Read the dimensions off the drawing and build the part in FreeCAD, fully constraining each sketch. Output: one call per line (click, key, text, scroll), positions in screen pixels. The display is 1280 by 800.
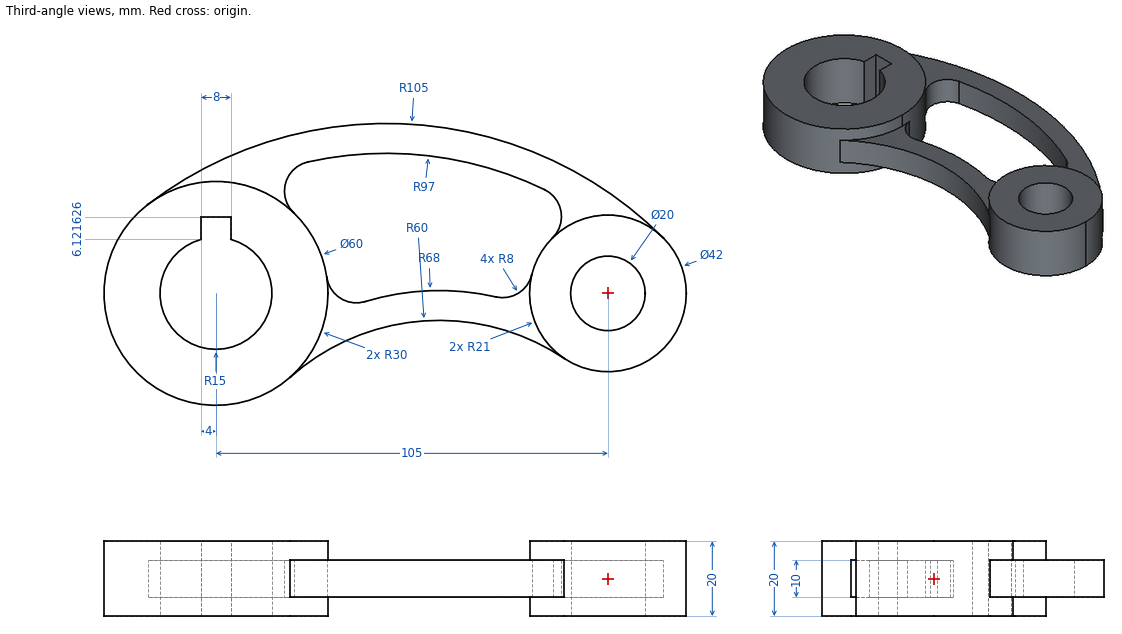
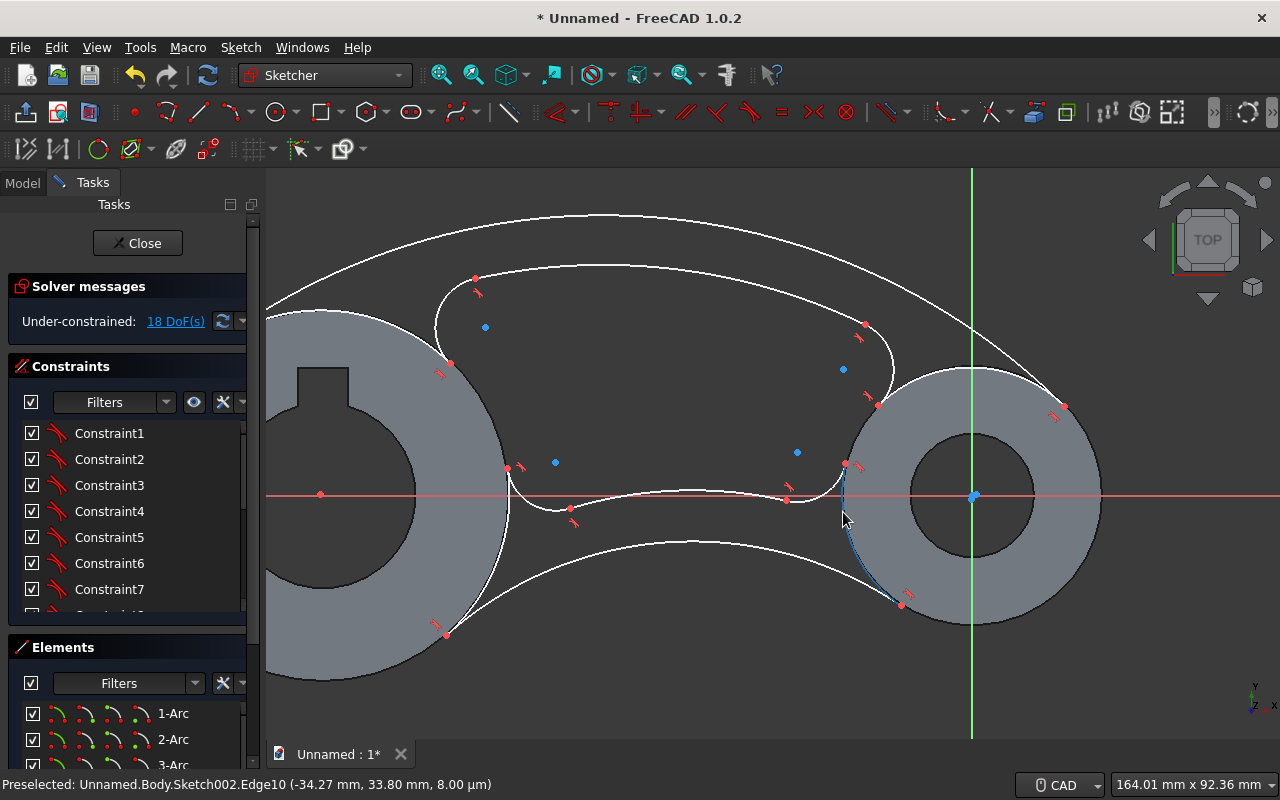
click(843, 512)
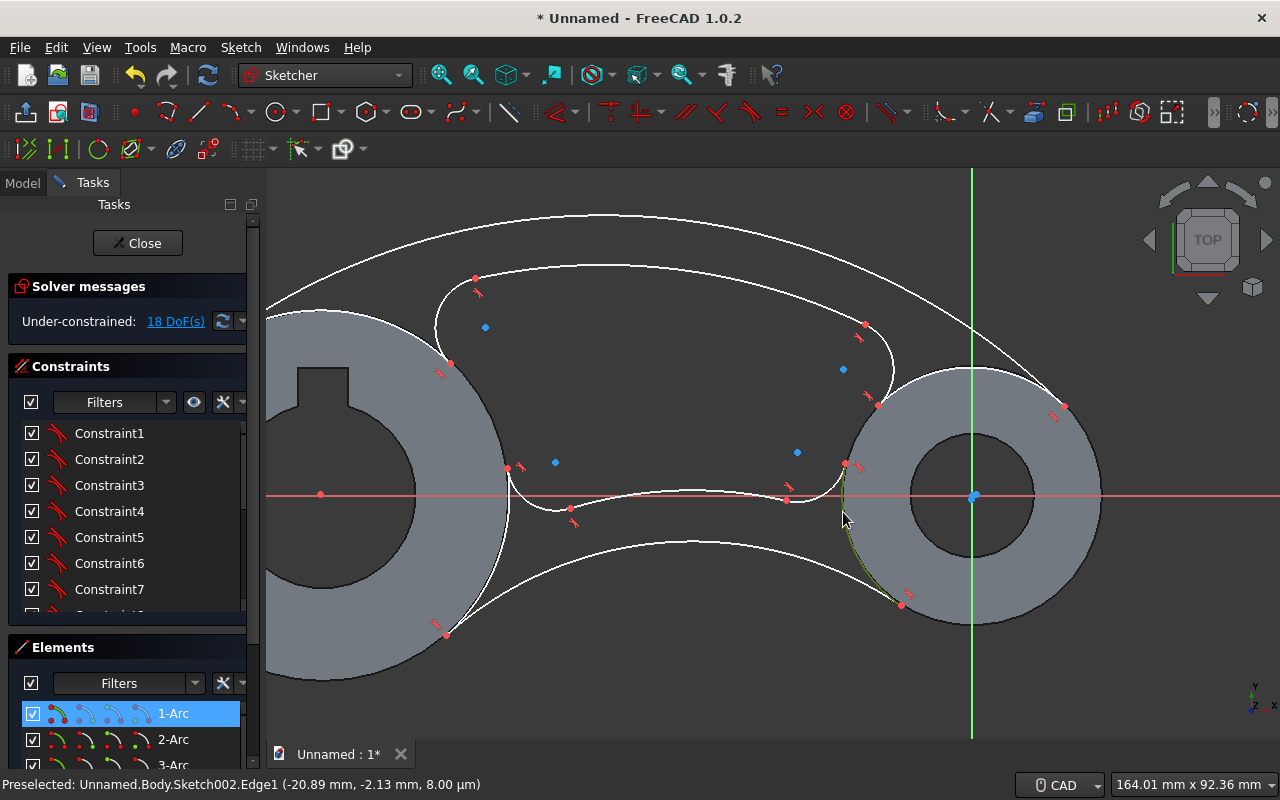
click(1012, 374)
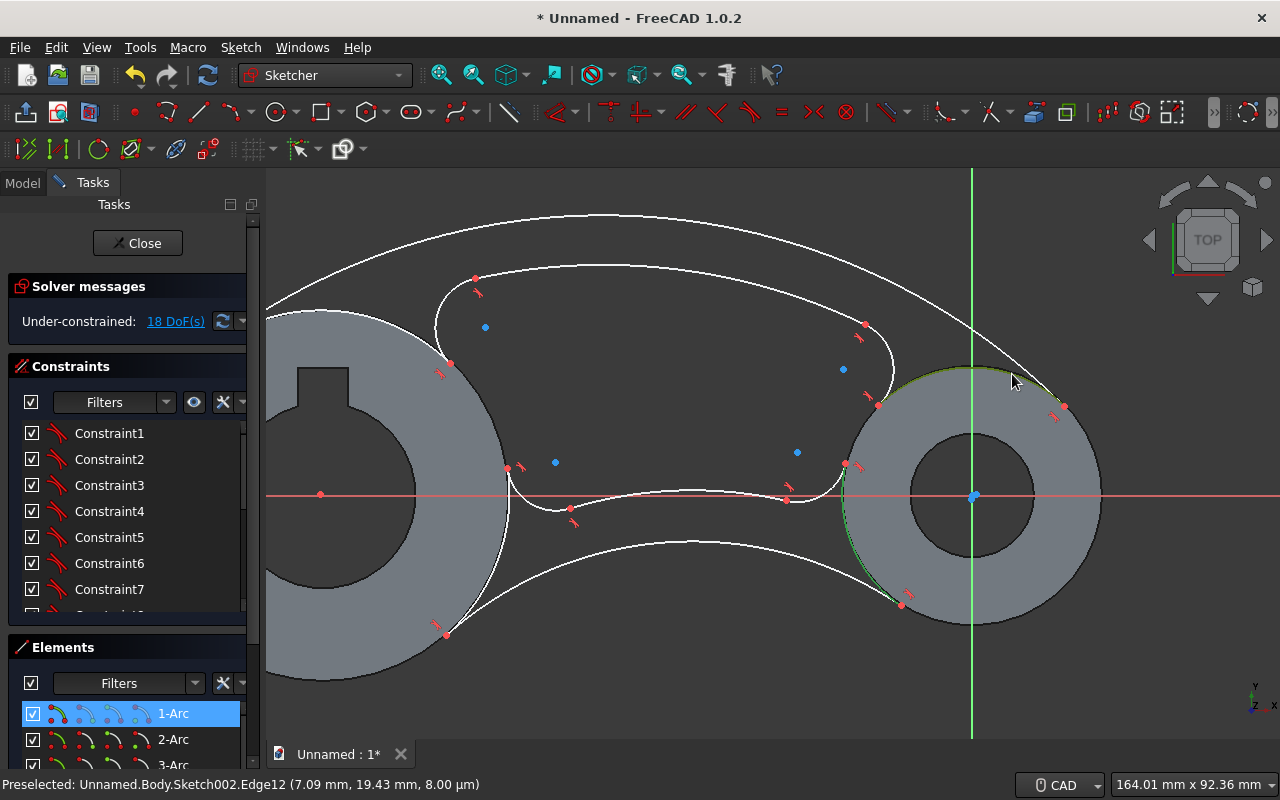
key(c)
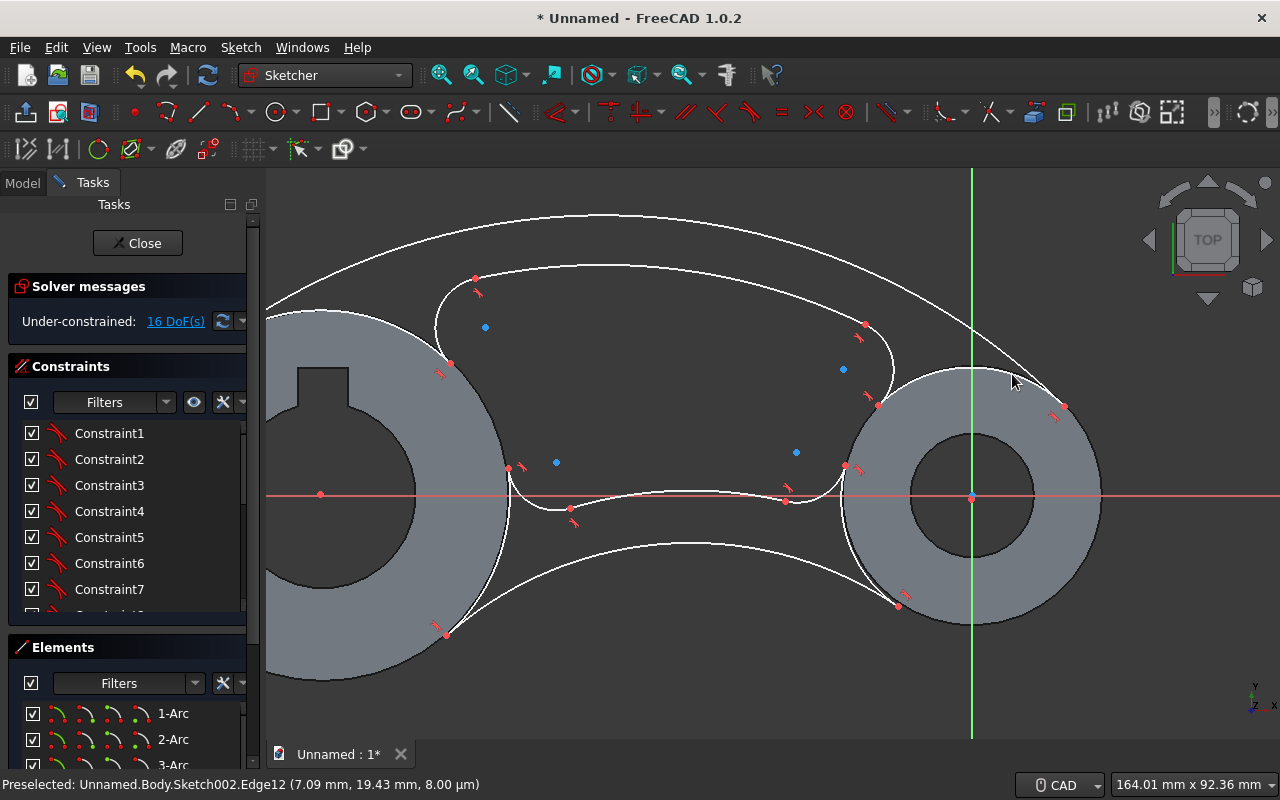
drag(961, 486, 982, 509)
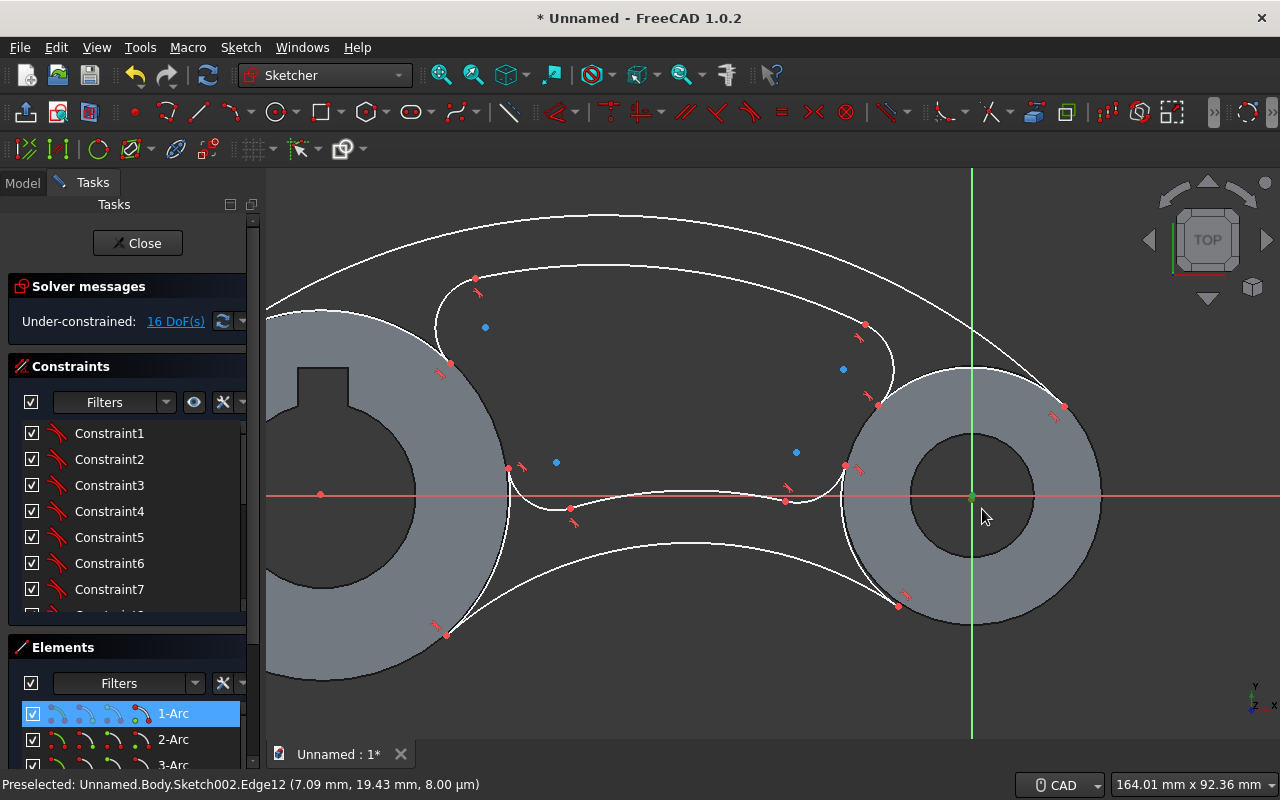
key(c)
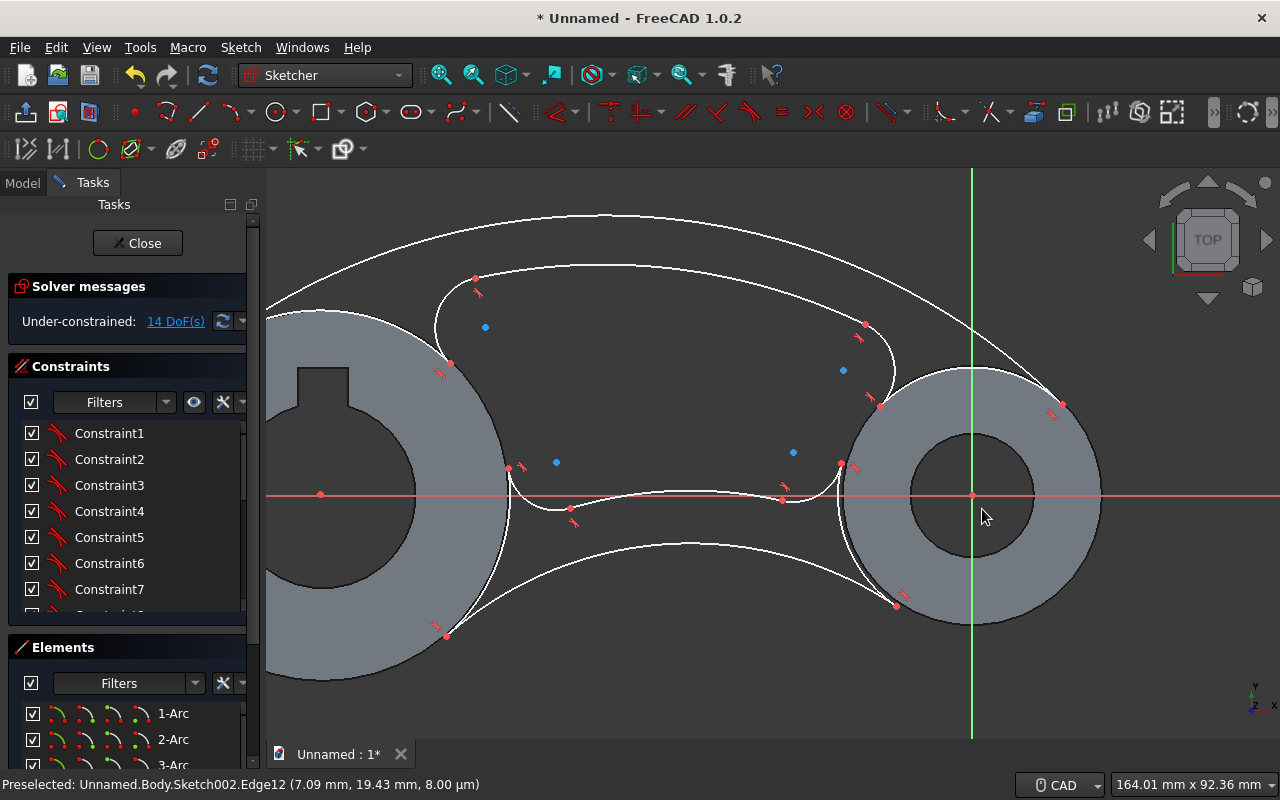
click(820, 494)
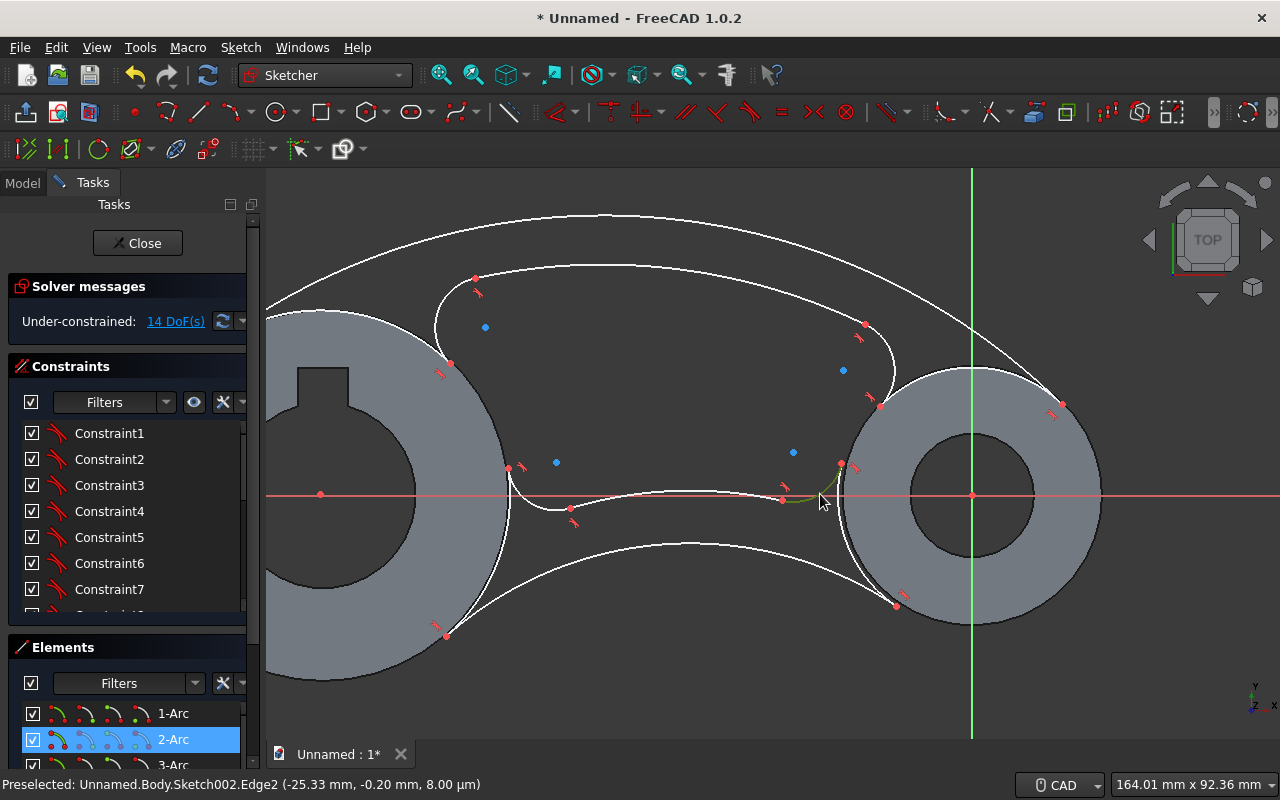
click(545, 509)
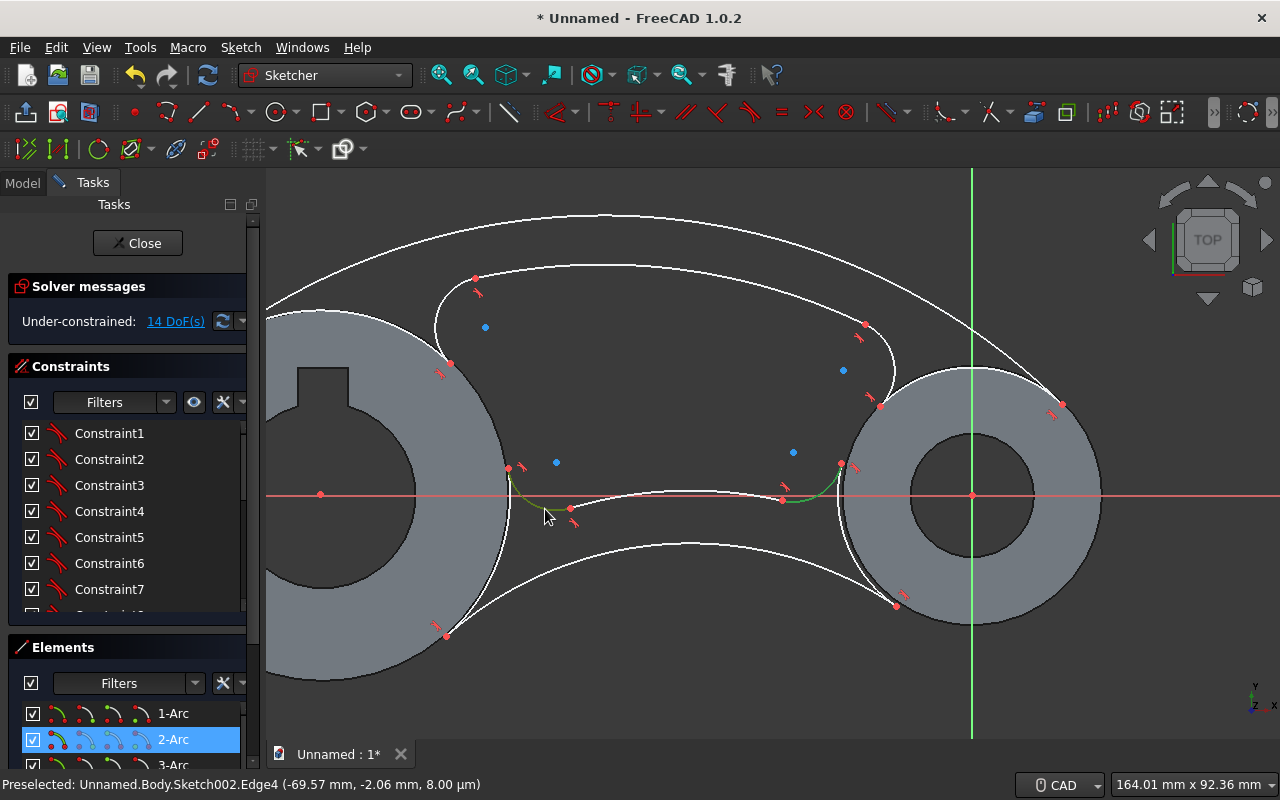
click(448, 295)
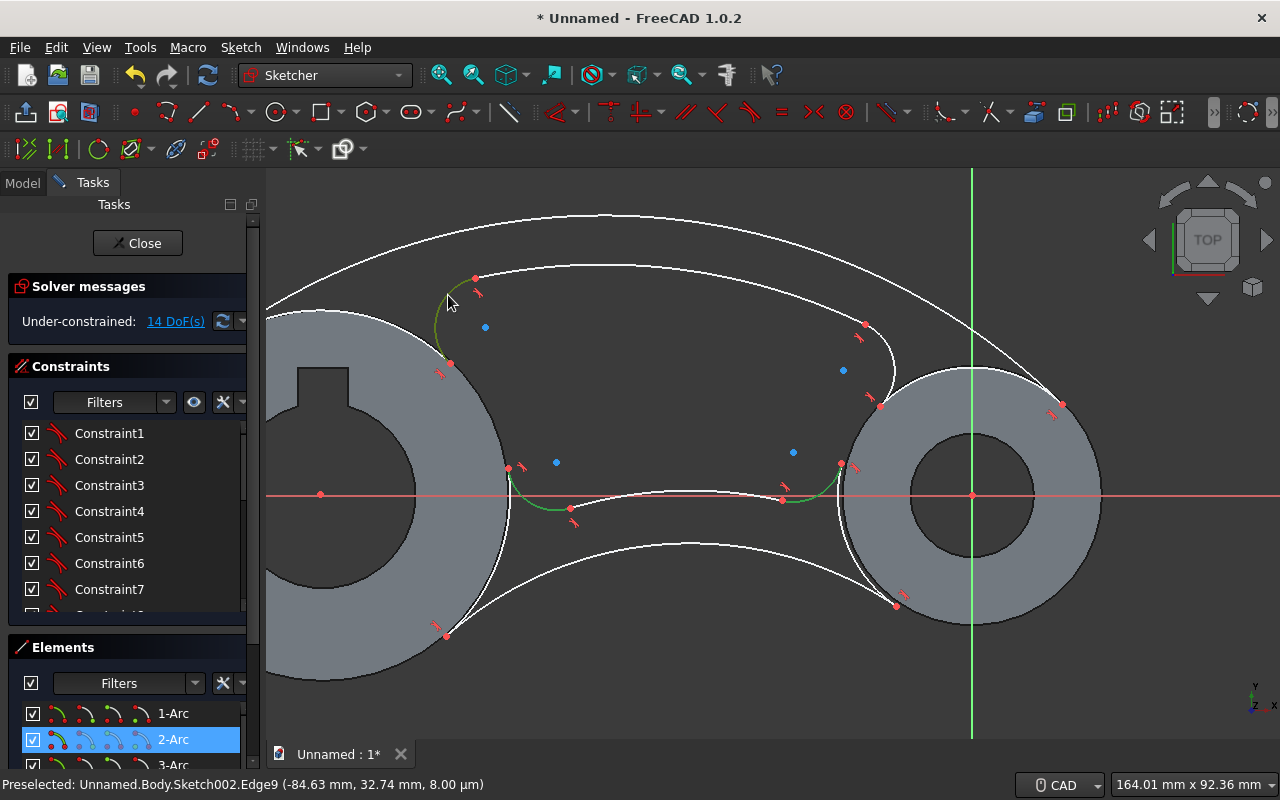
scroll(894, 381, up, 2)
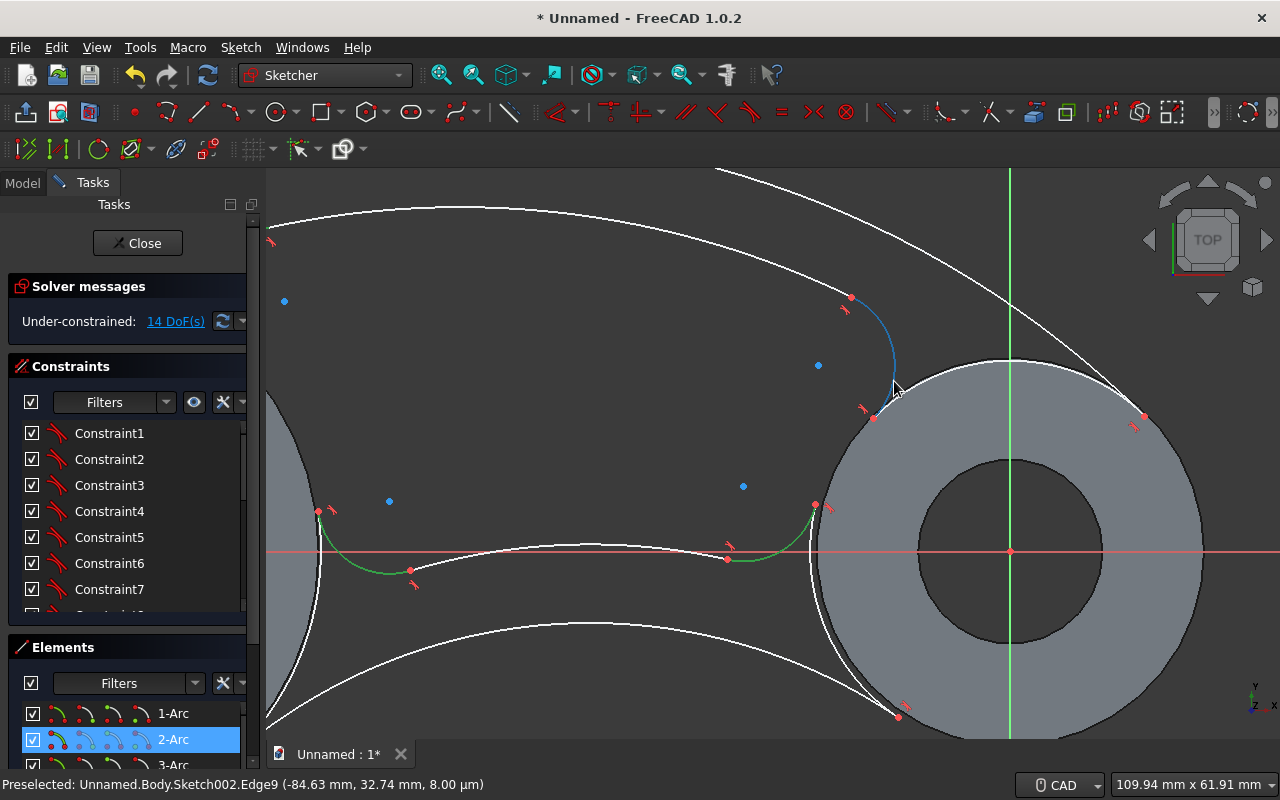
click(893, 381)